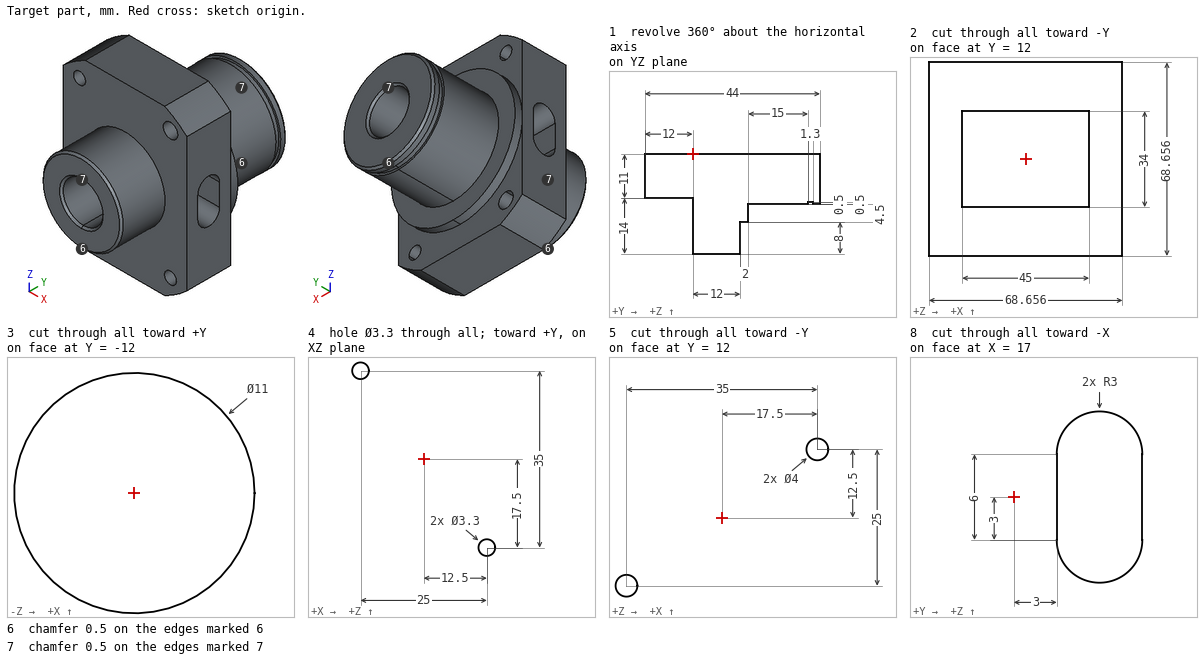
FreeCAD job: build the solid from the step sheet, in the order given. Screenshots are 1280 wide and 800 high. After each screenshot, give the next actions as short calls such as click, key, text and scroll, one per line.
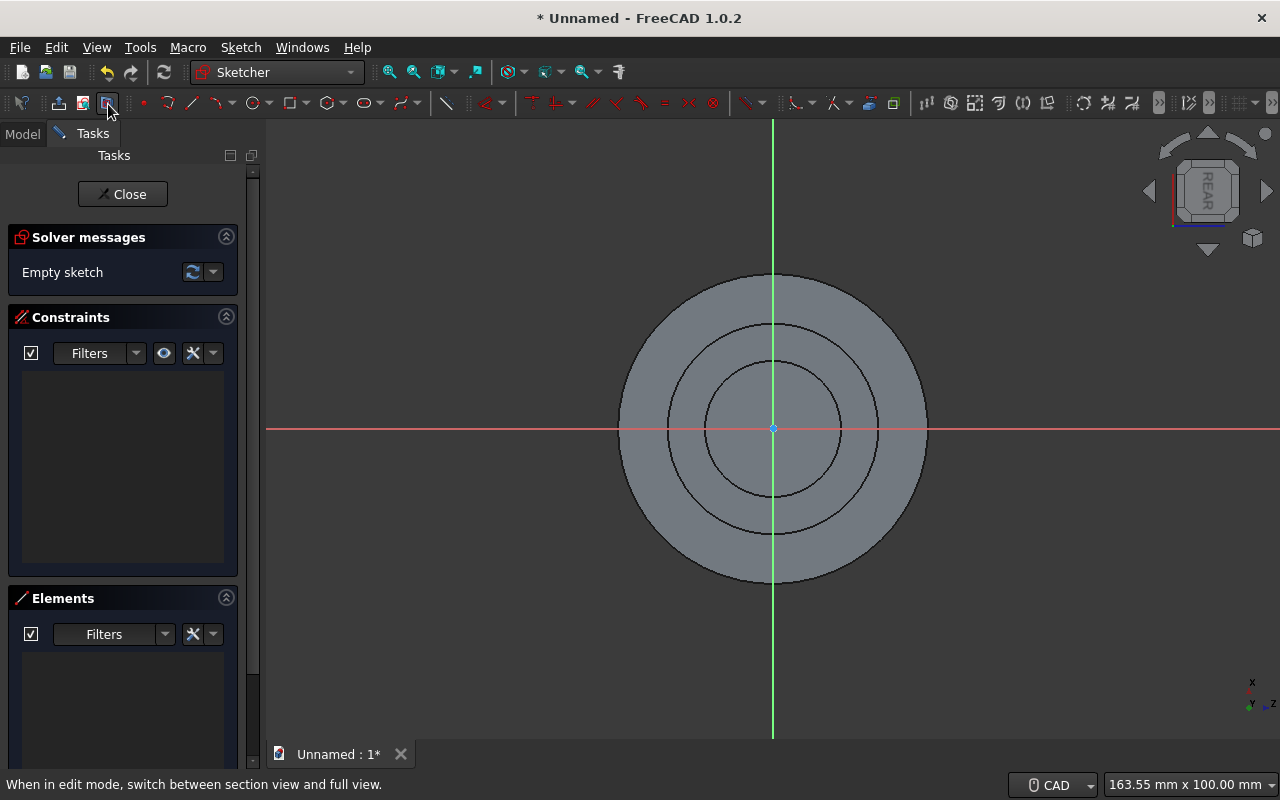
click(308, 104)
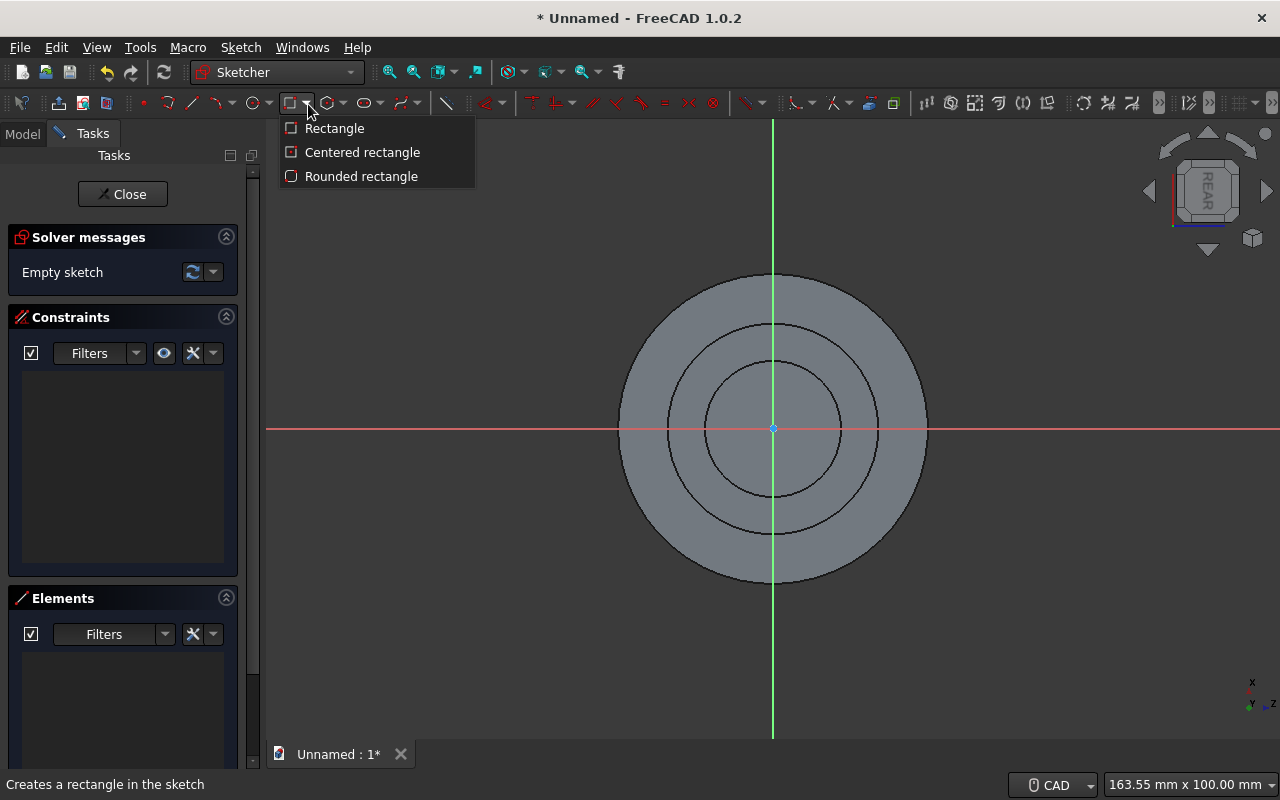
click(378, 152)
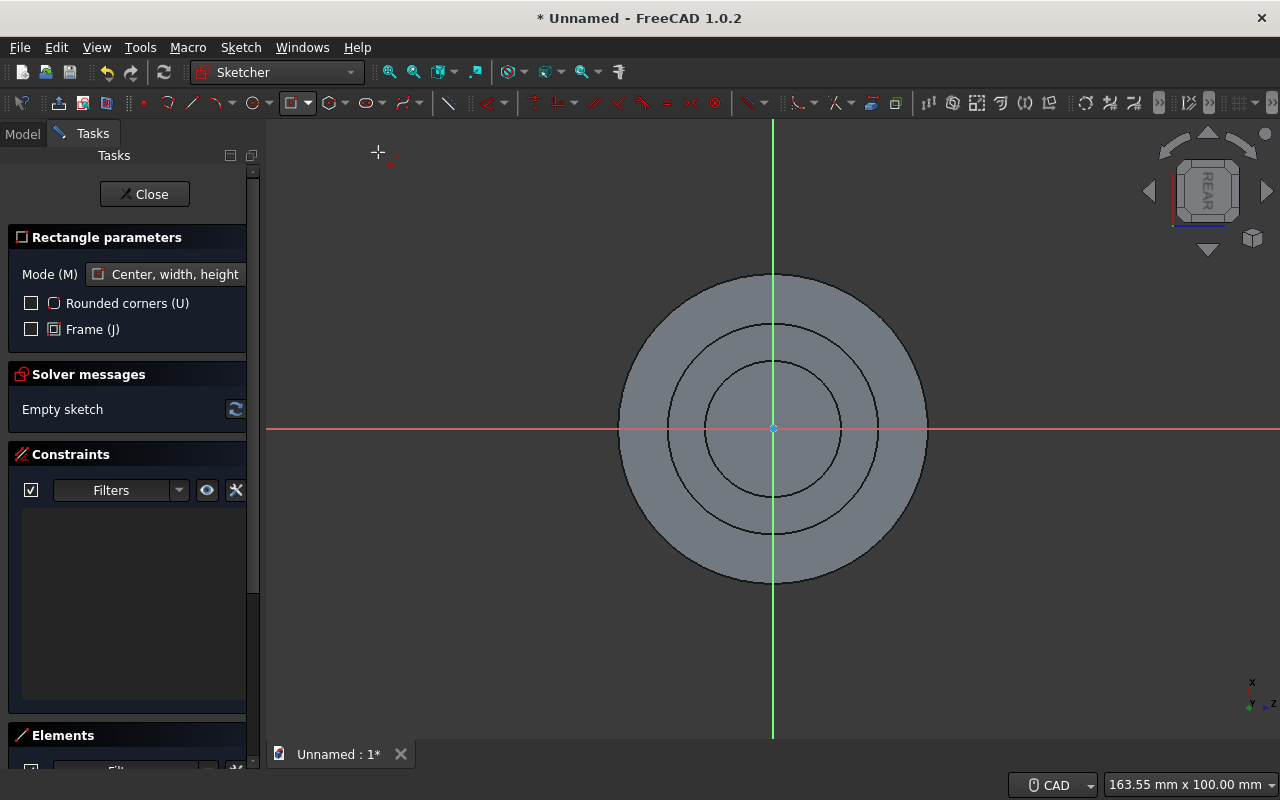
click(773, 429)
move(986, 216)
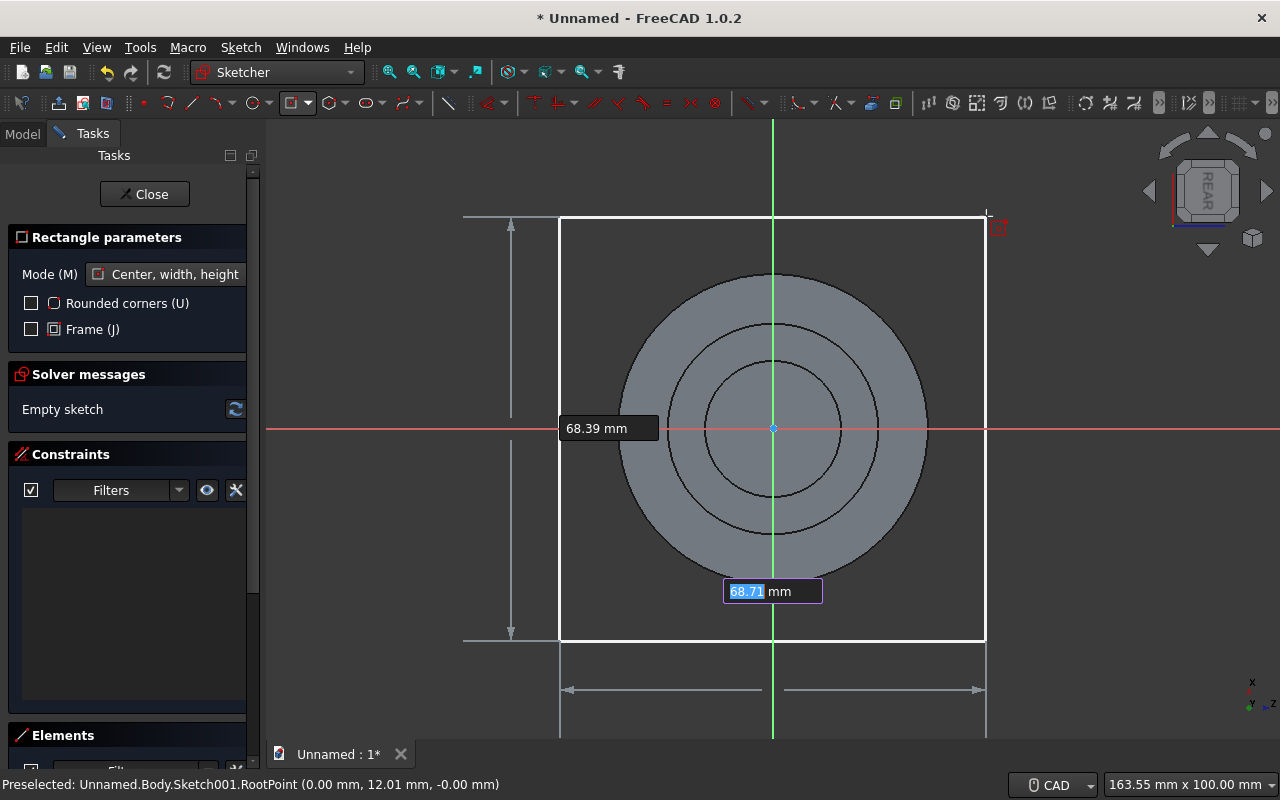
text(68.656)
key(Tab)
text(68.656)
key(Return)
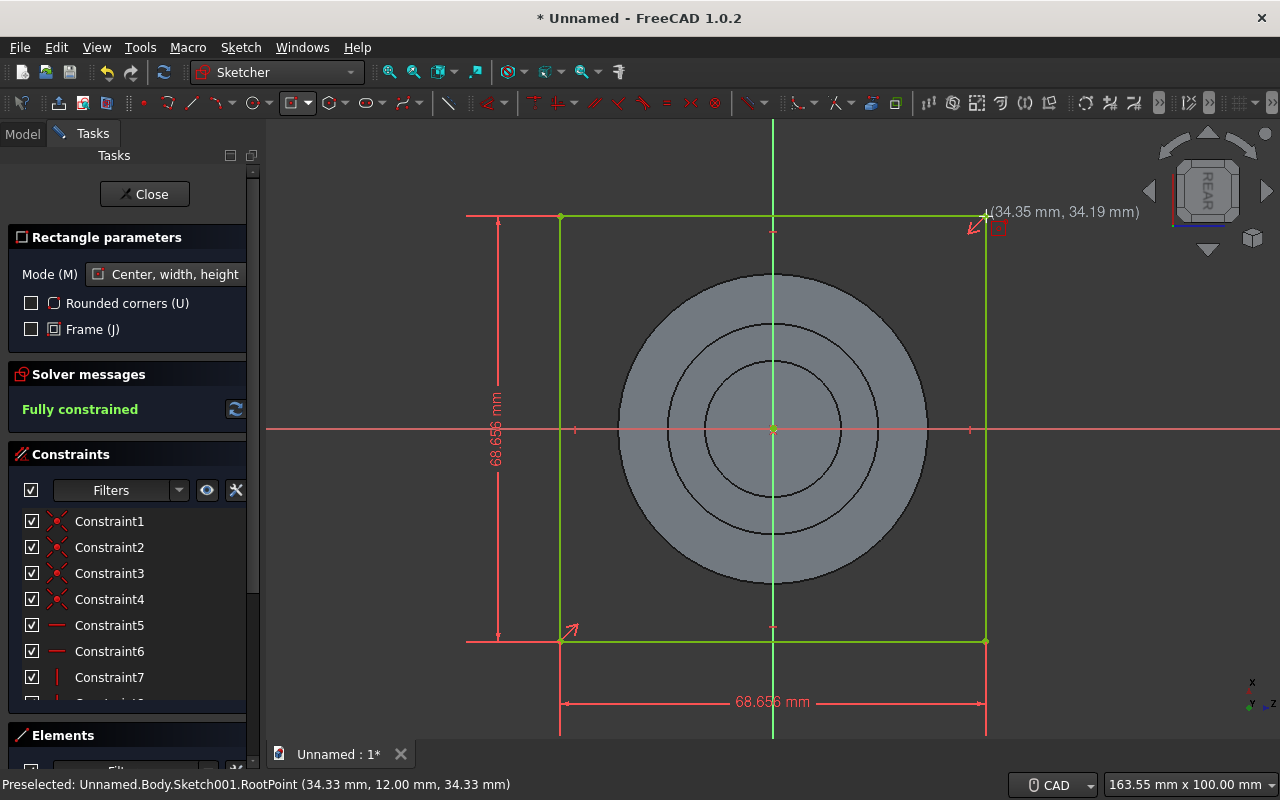
click(773, 429)
move(913, 324)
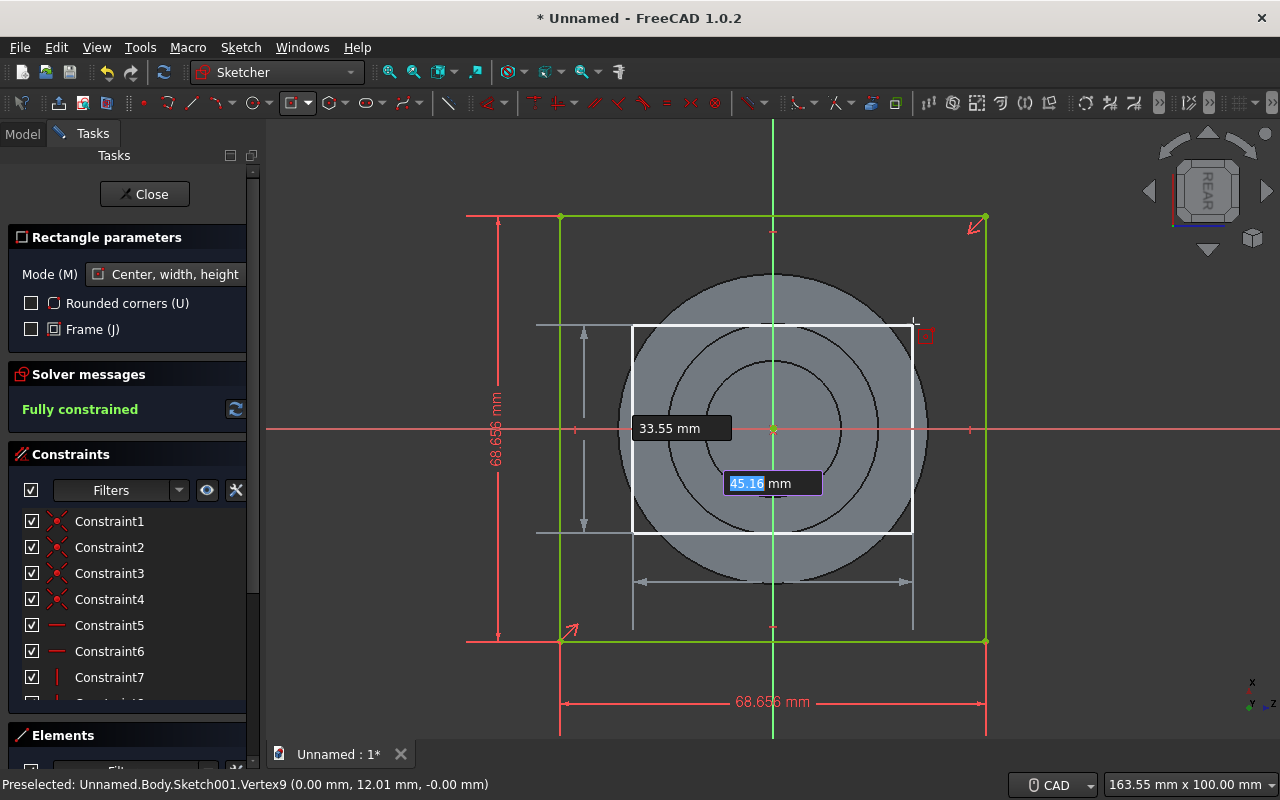
text(45)
key(Tab)
text(34)
key(Return)
key(Escape)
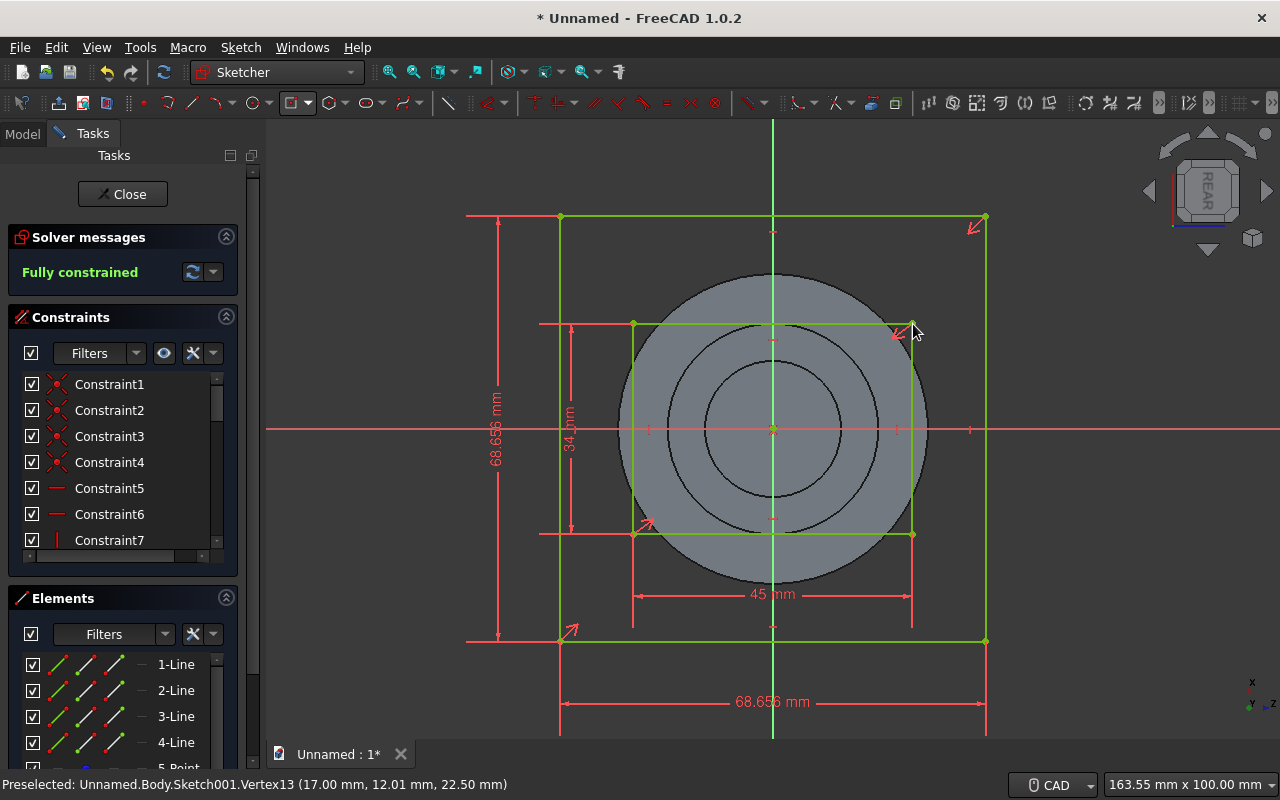
click(123, 194)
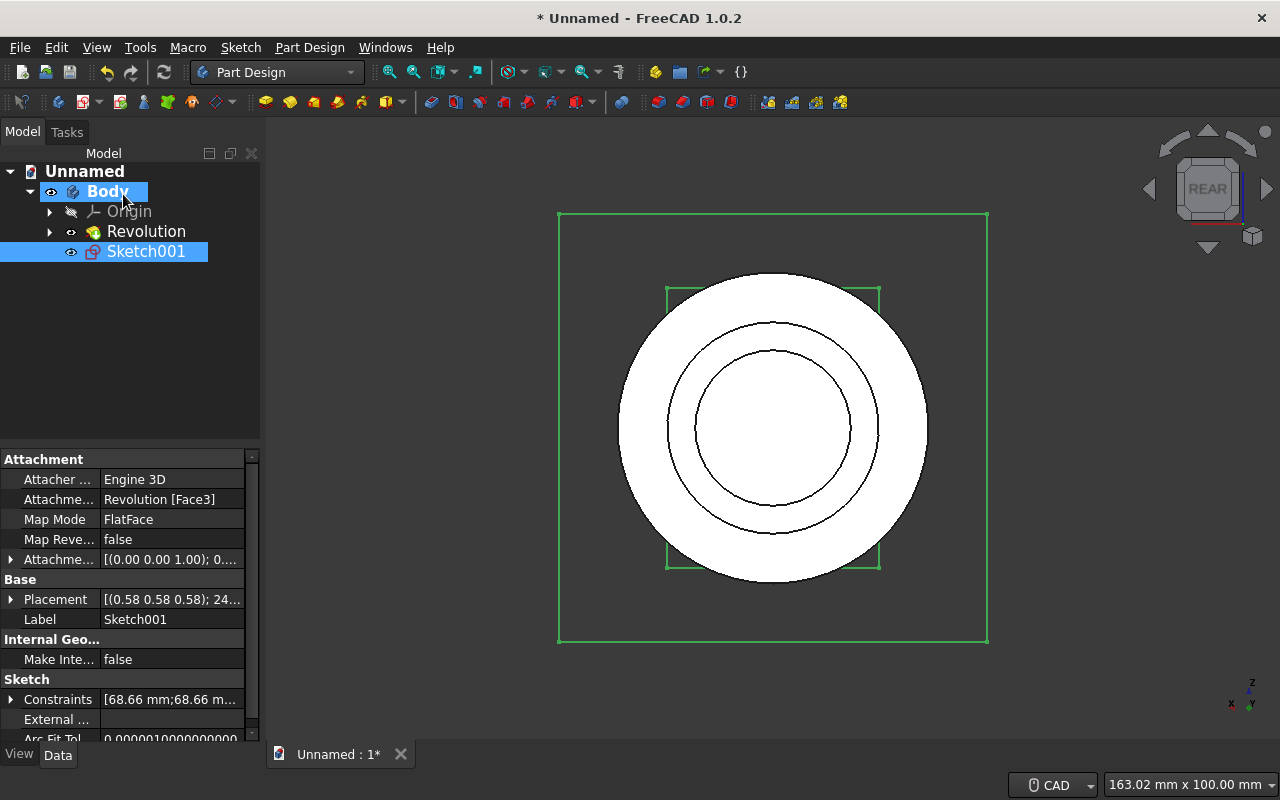
click(432, 102)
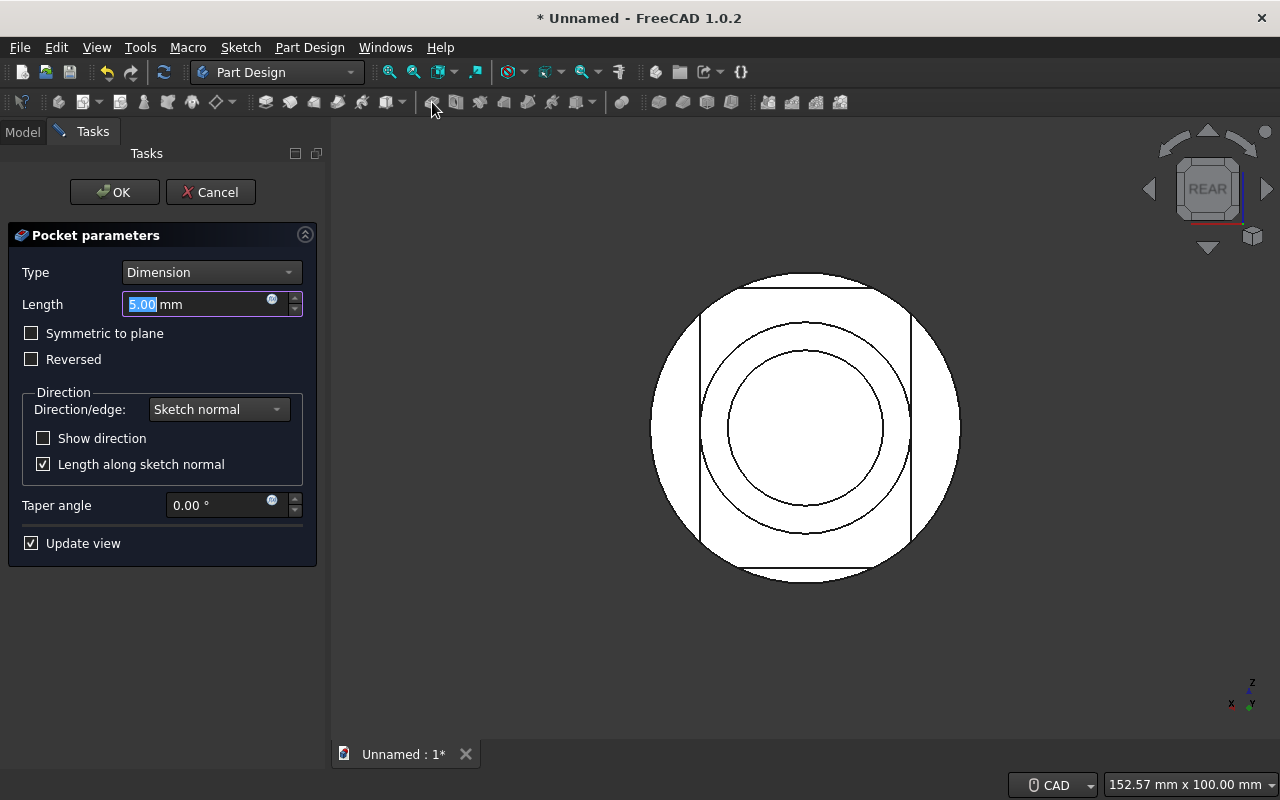
click(212, 272)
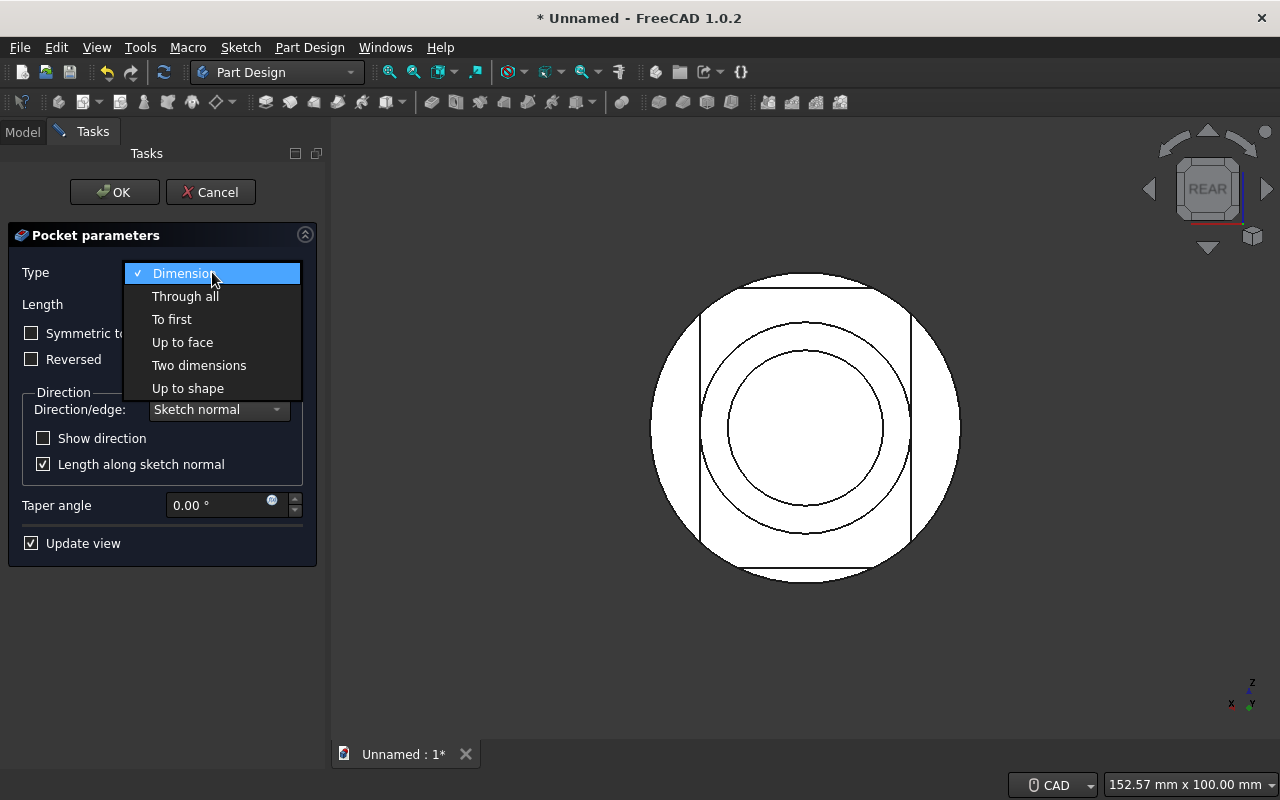
click(212, 296)